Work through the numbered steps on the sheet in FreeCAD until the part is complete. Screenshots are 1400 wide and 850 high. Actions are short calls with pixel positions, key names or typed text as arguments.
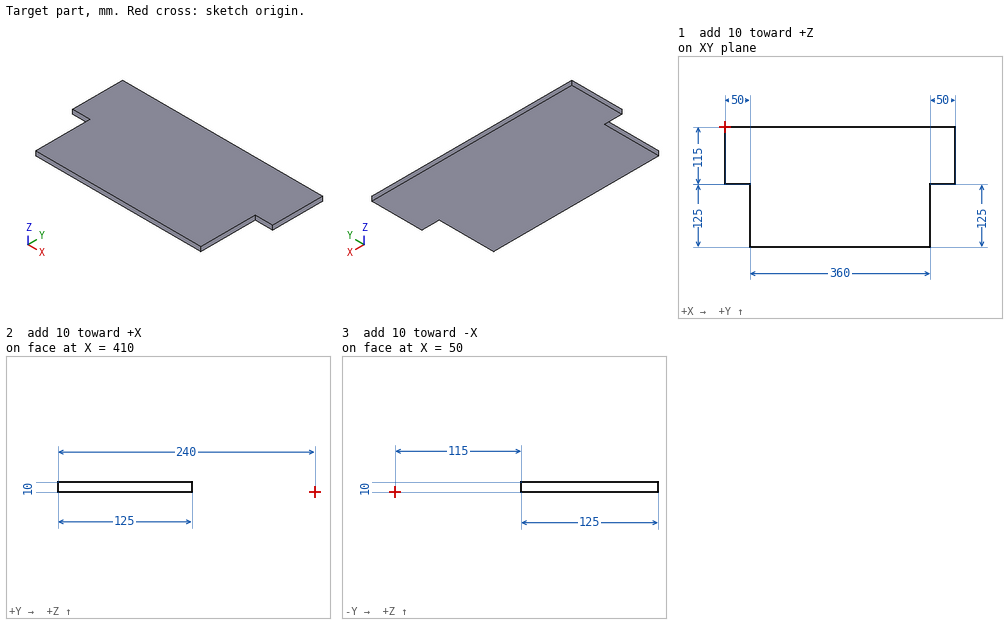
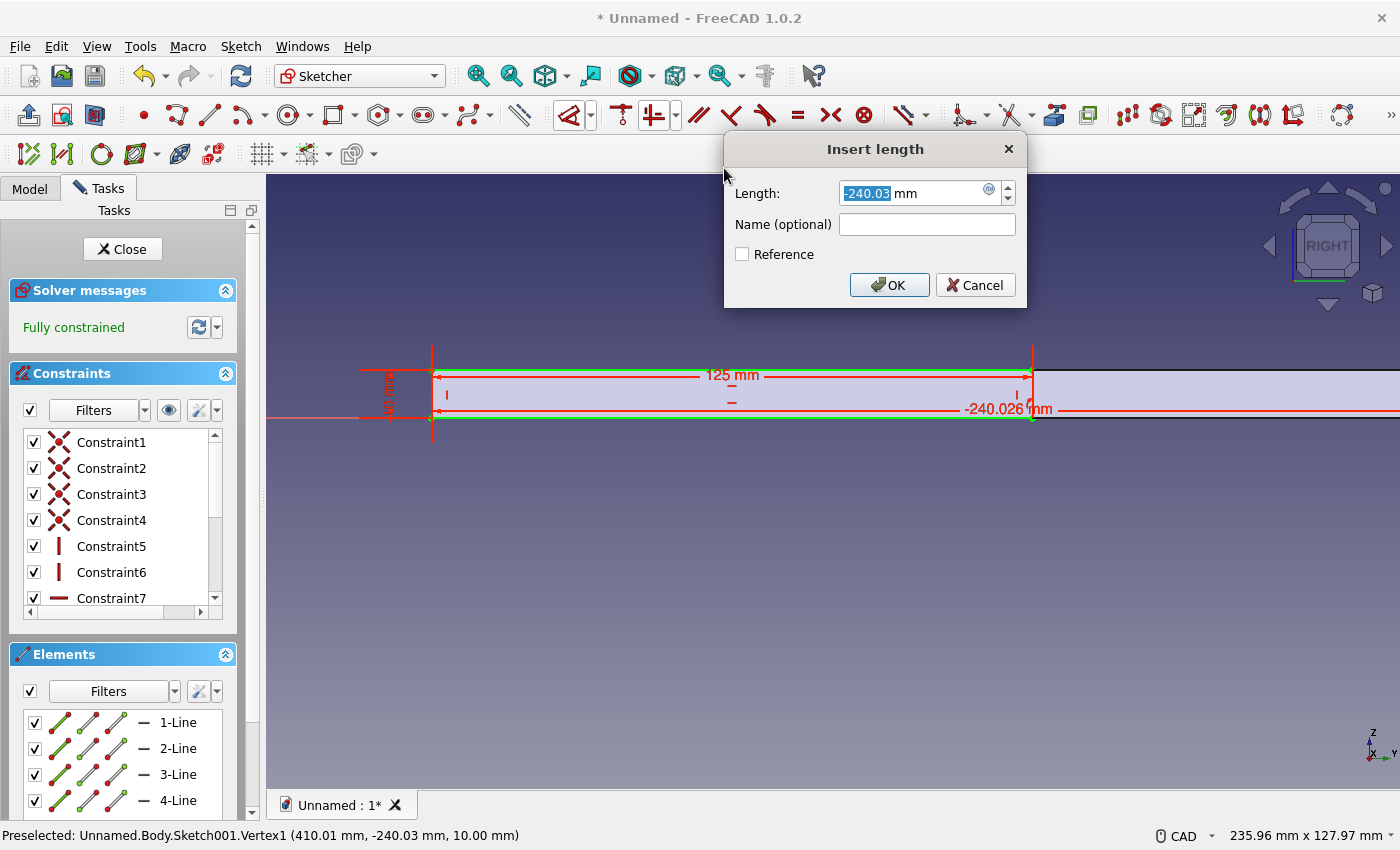
text(-240)
key(Return)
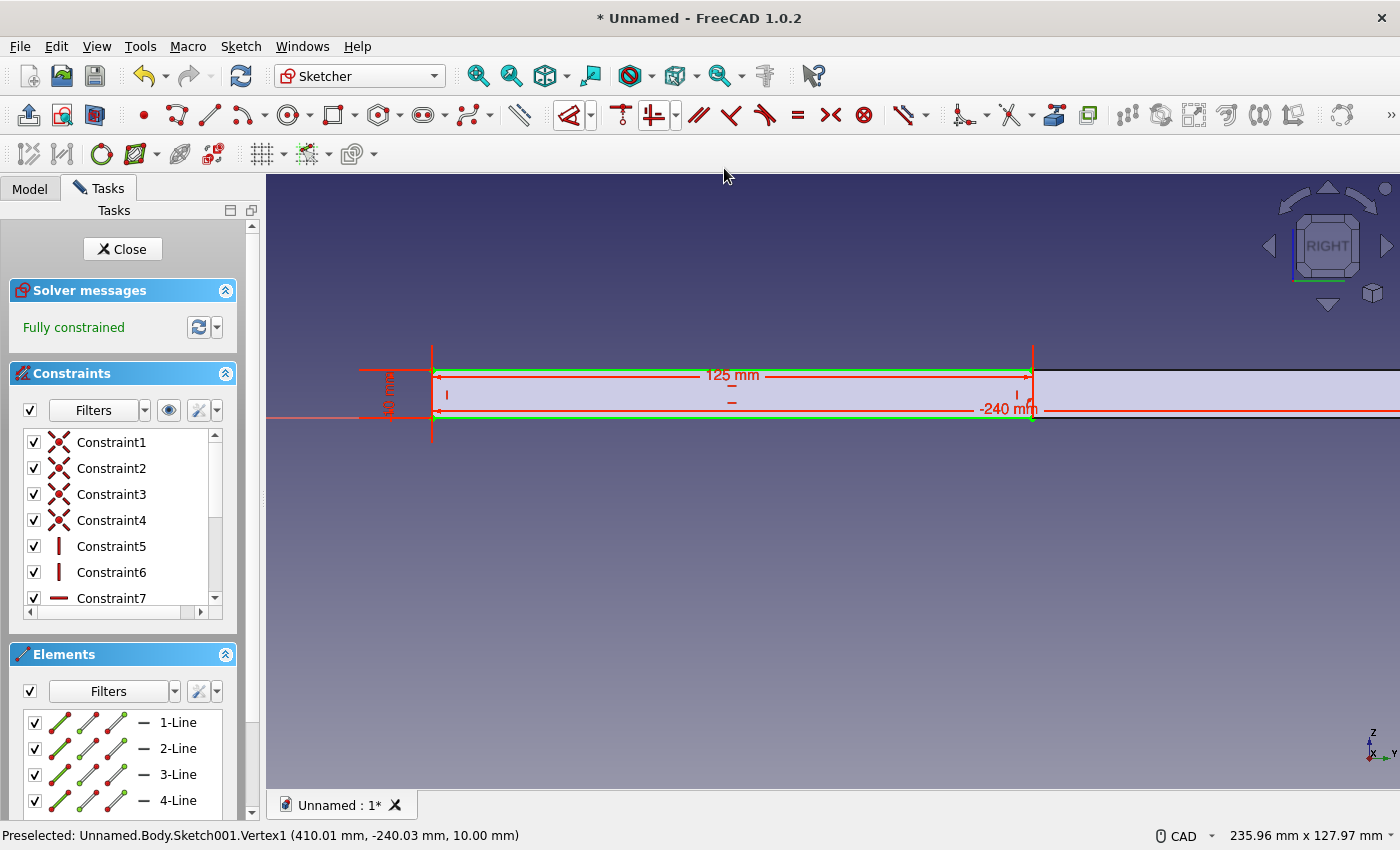
click(123, 249)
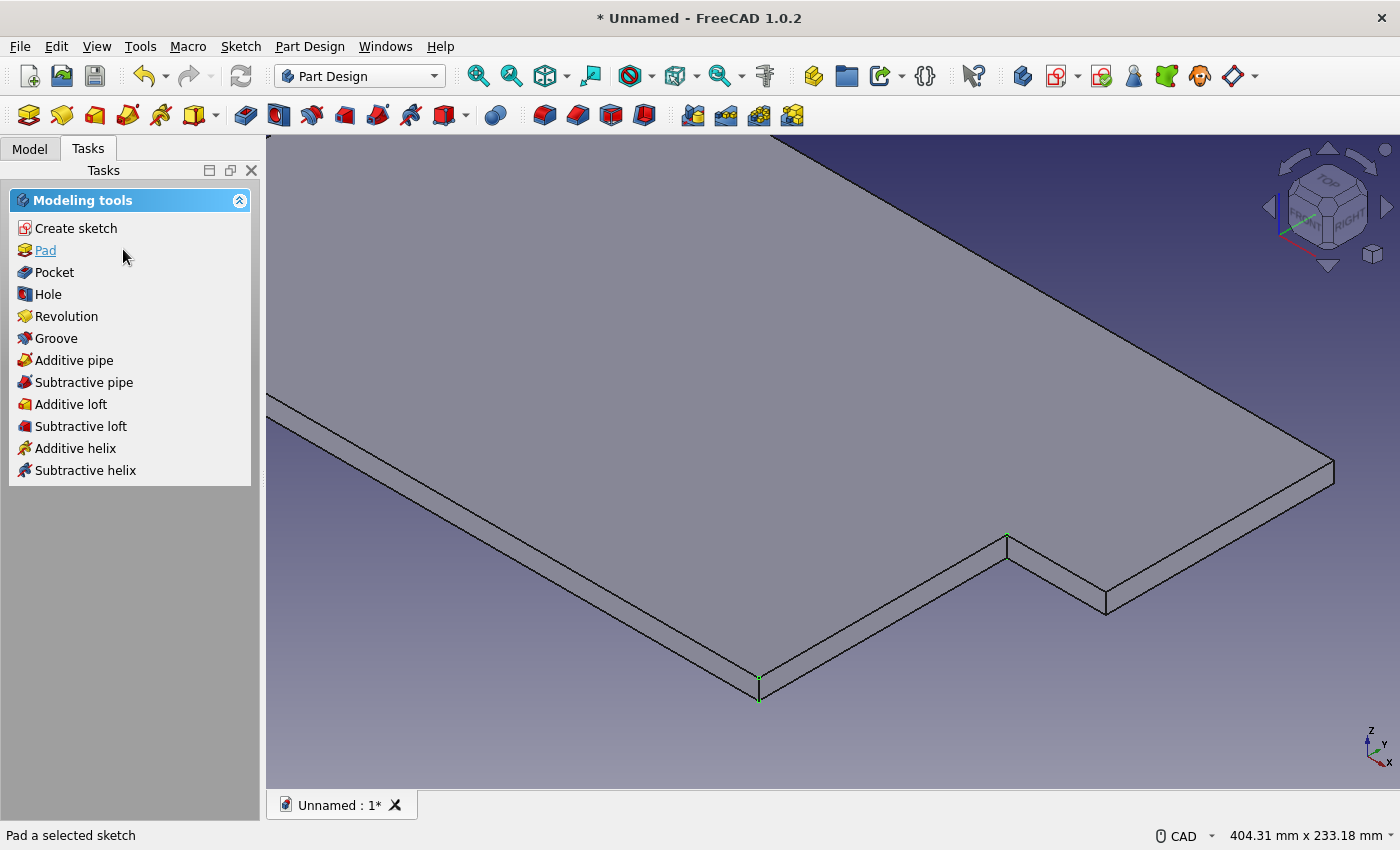
click(29, 116)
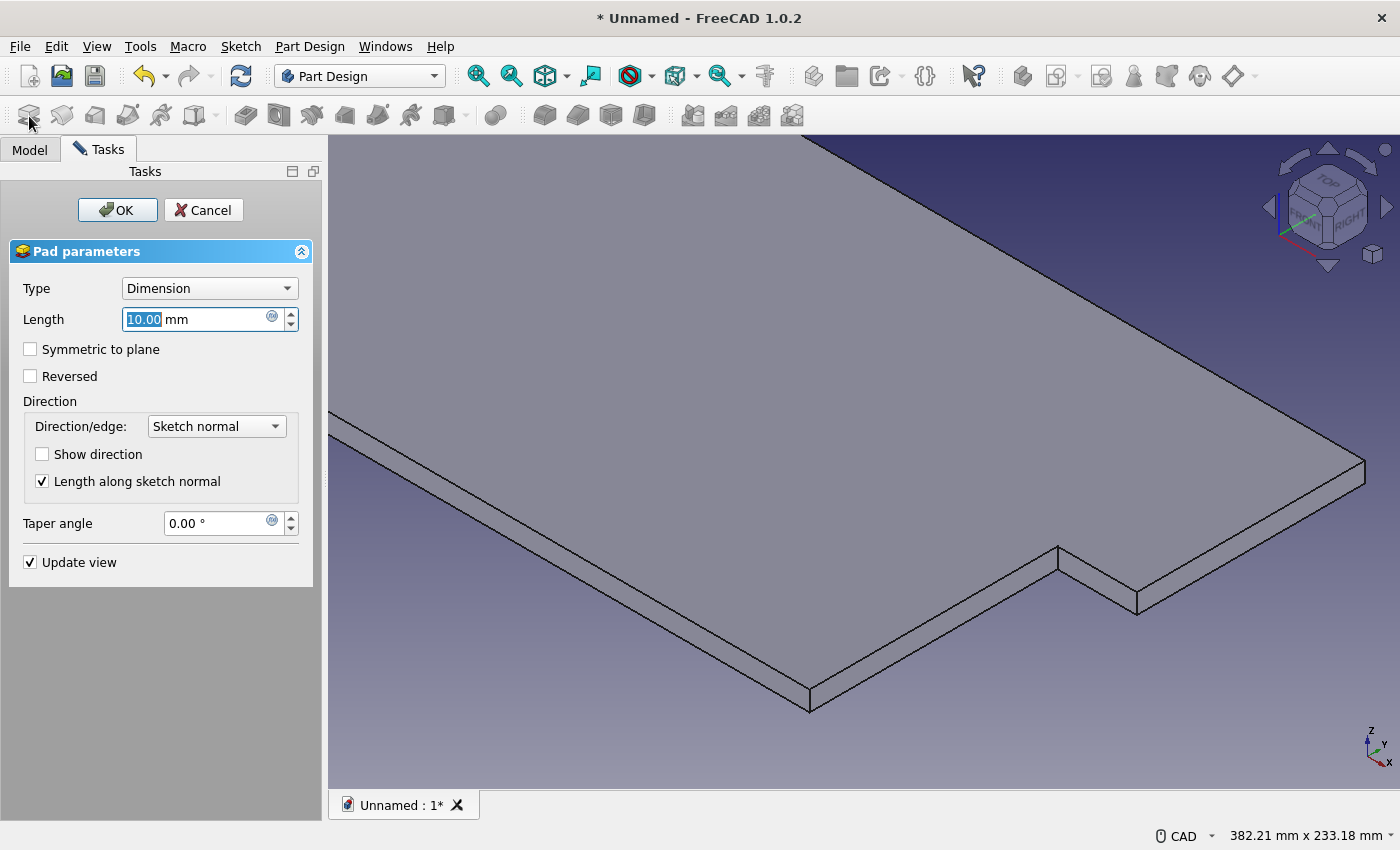
text(10)
key(Tab)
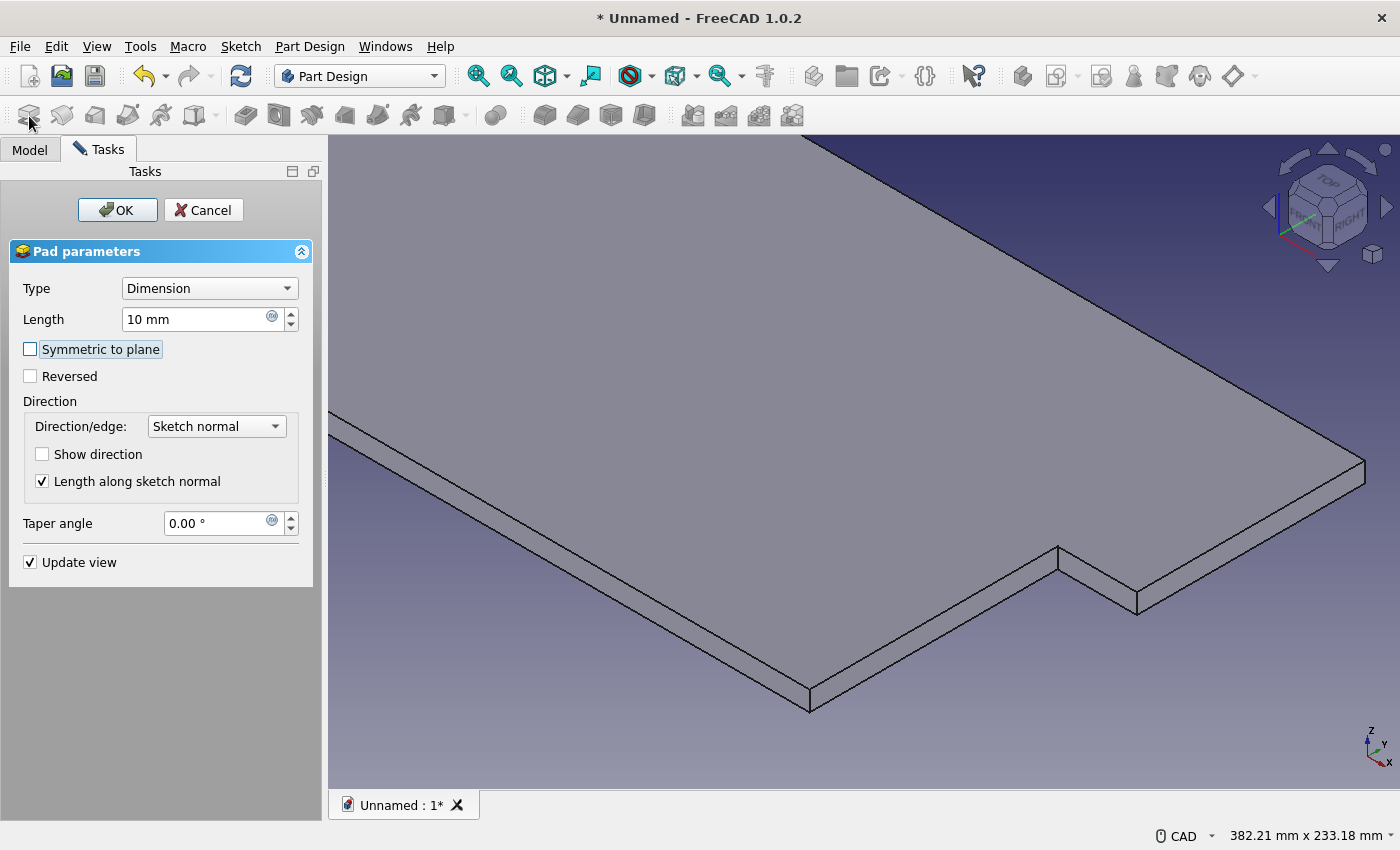
click(118, 210)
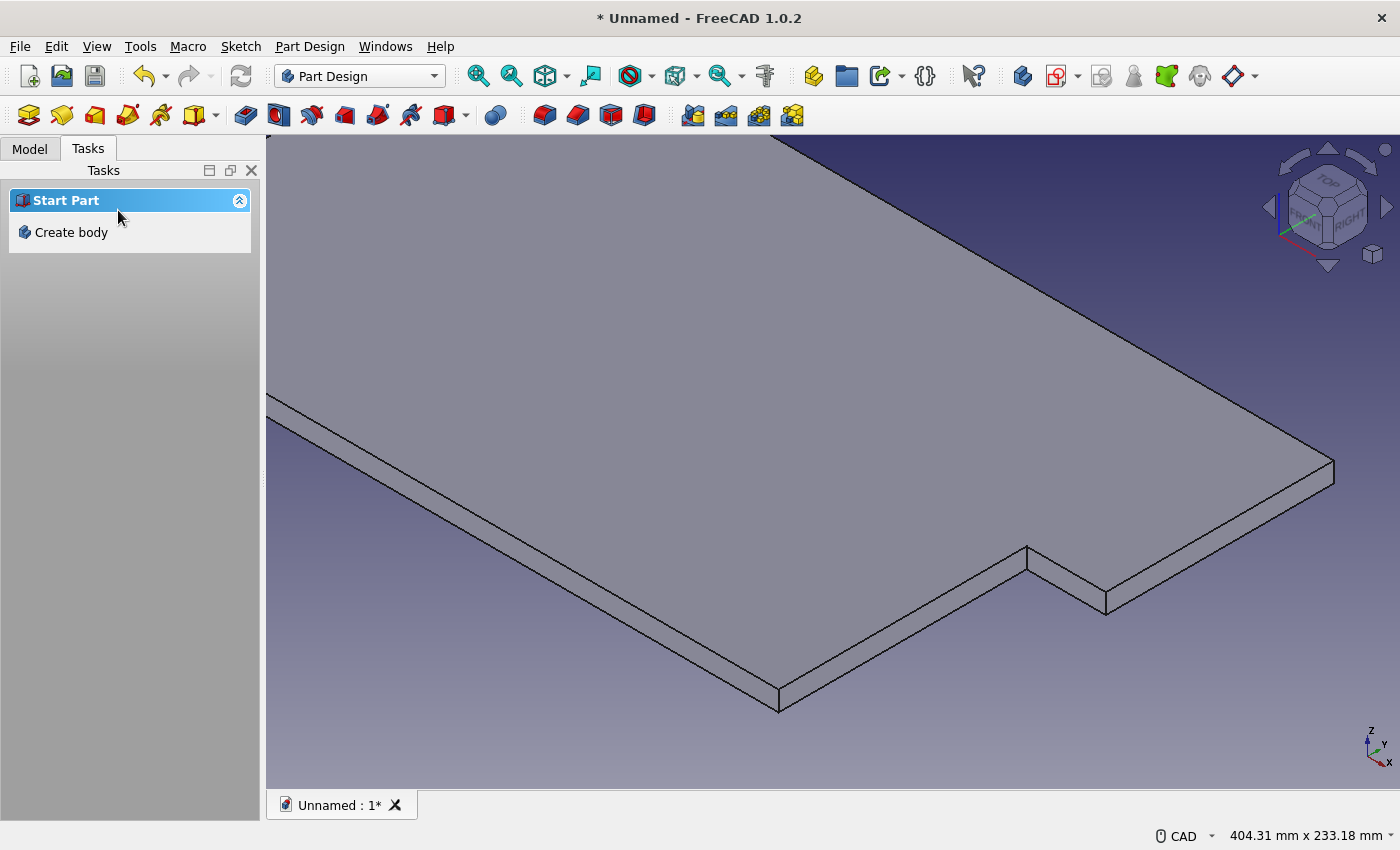
click(479, 76)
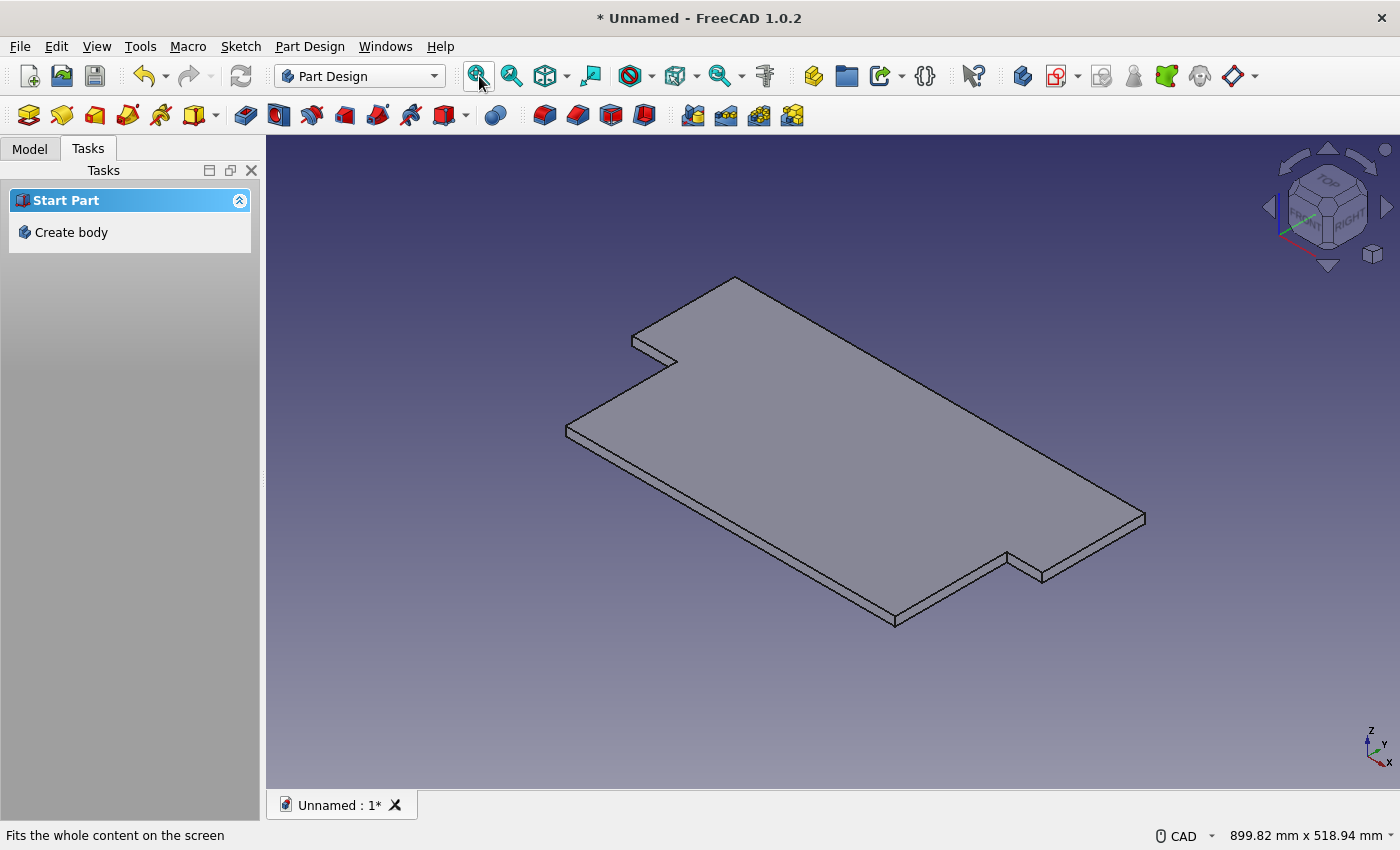
key(6)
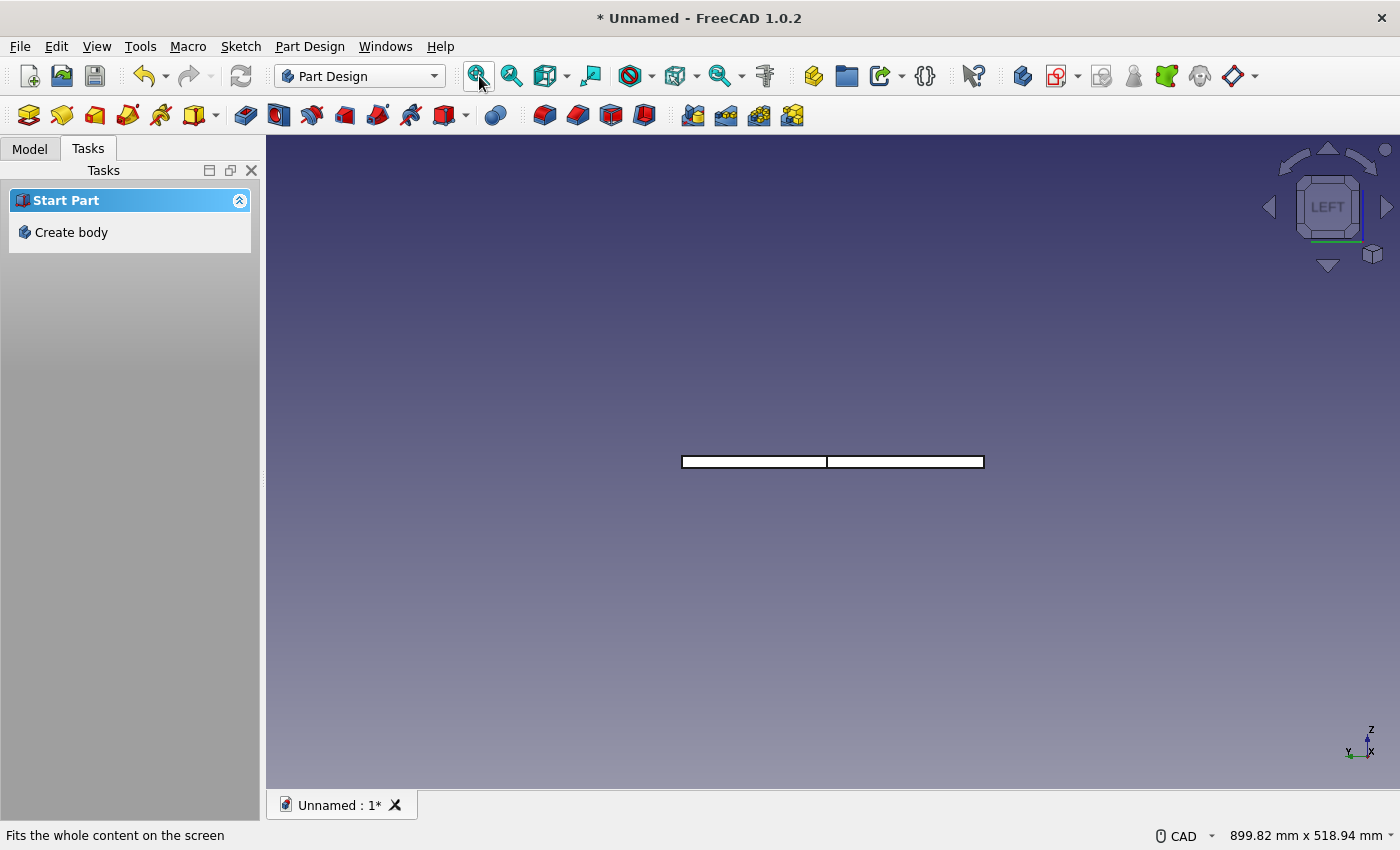
click(479, 76)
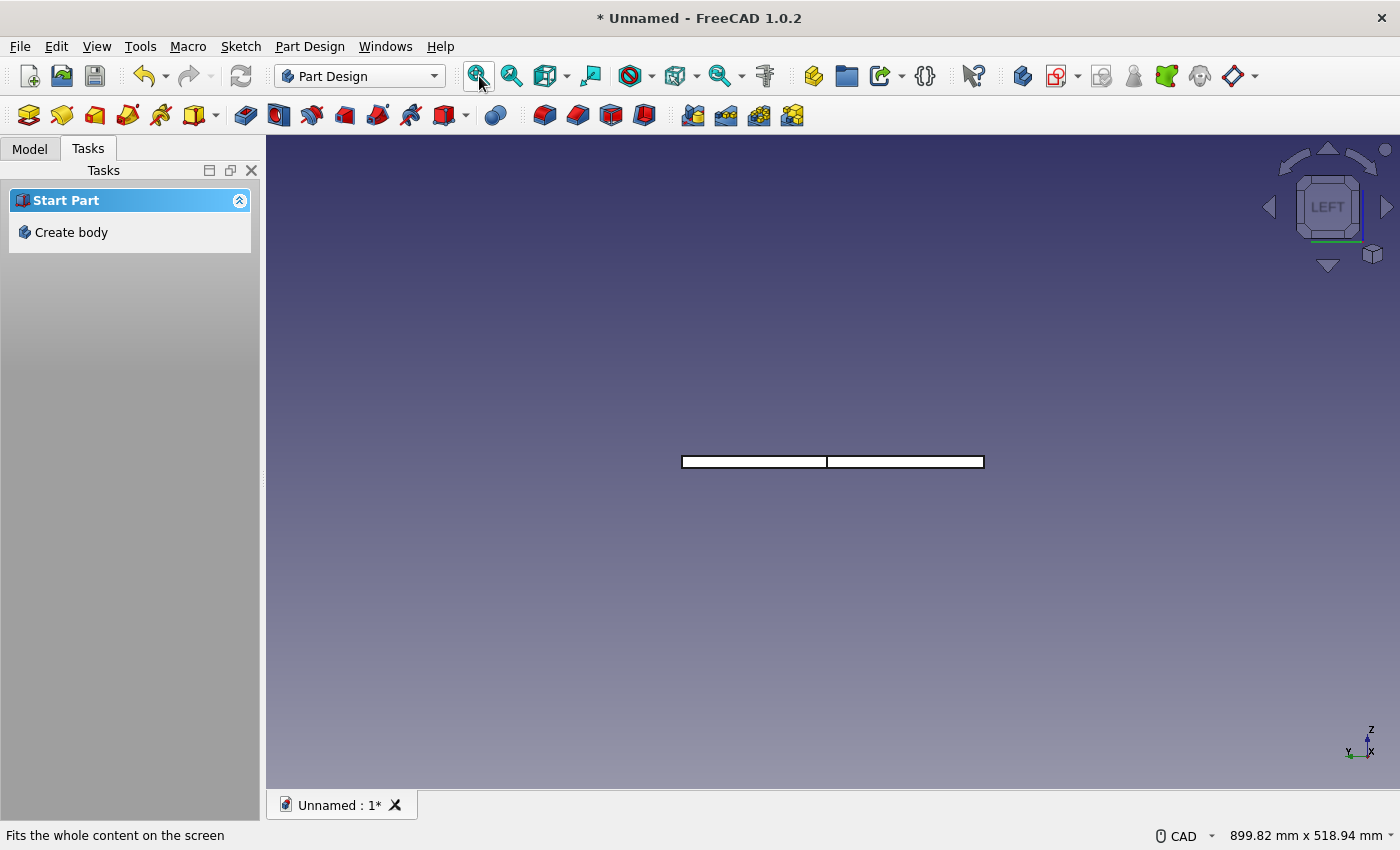
scroll(838, 461, up, 4)